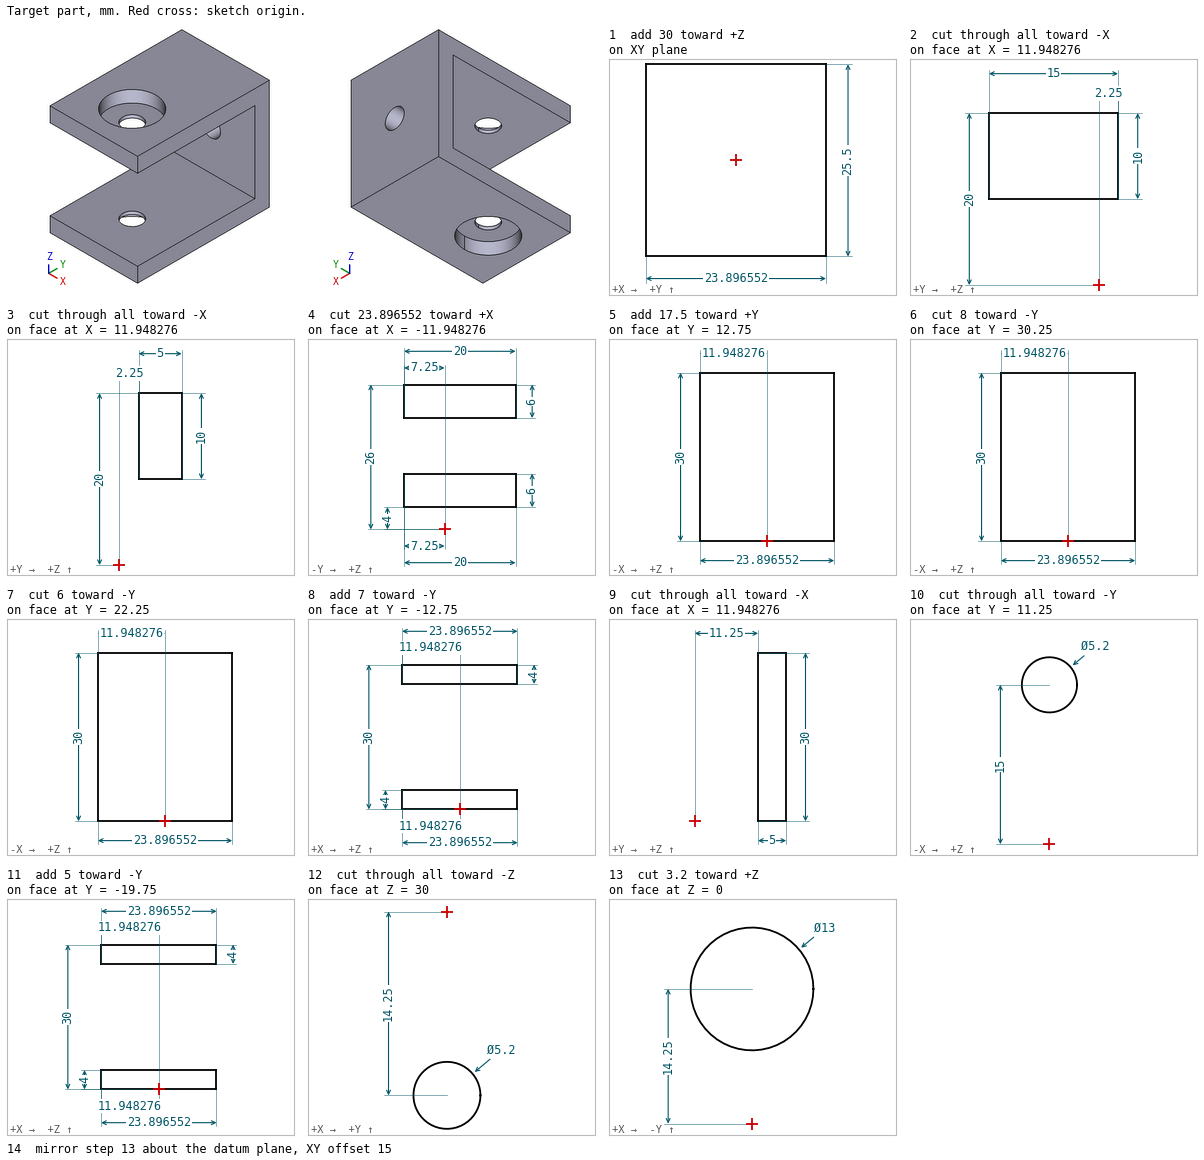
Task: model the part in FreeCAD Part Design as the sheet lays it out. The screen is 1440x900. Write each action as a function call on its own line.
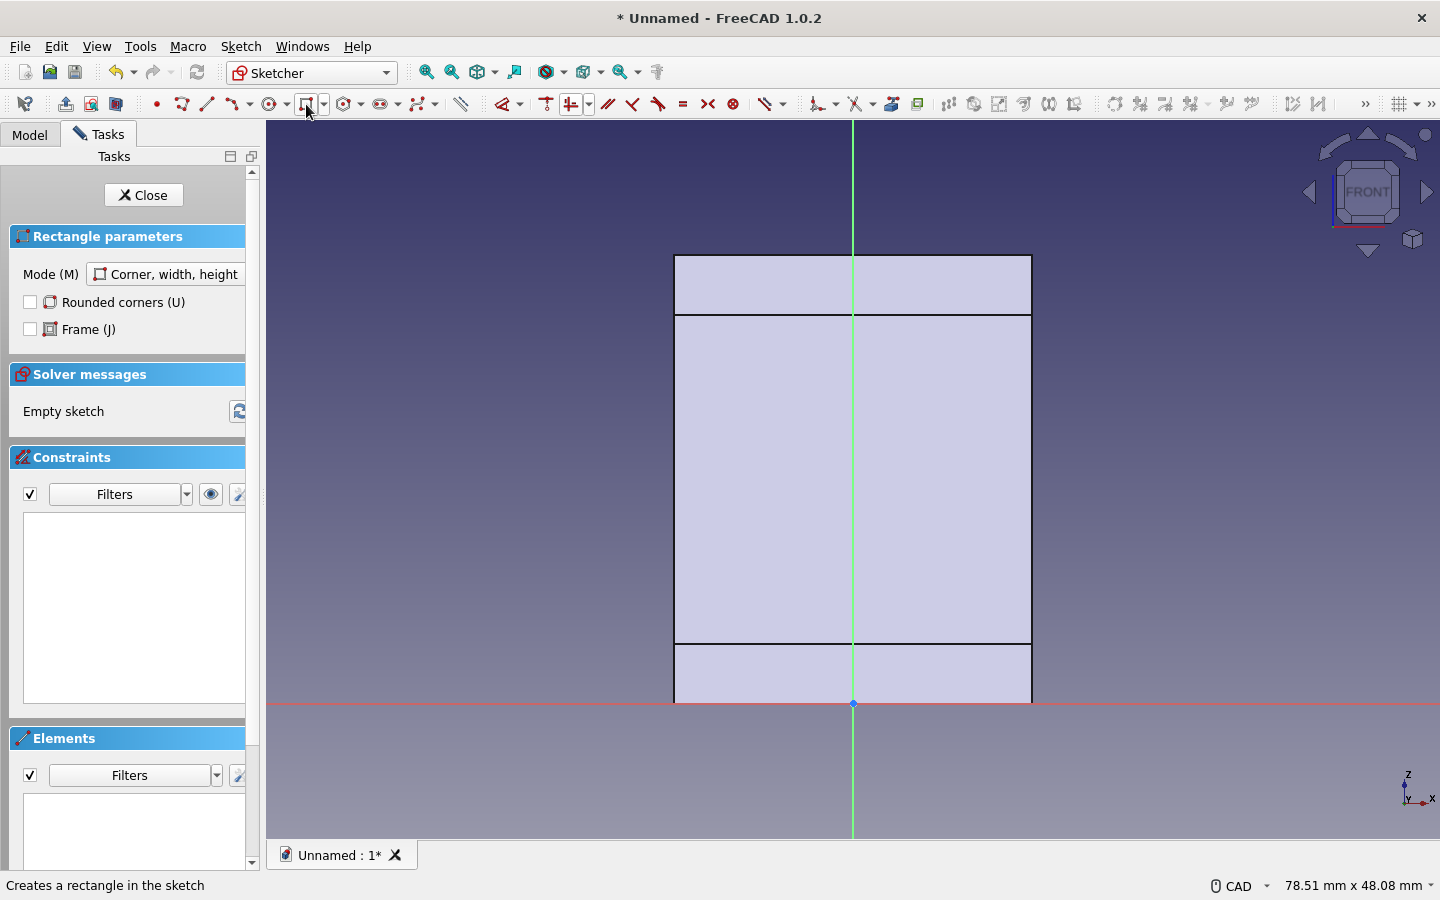
click(674, 255)
move(1032, 315)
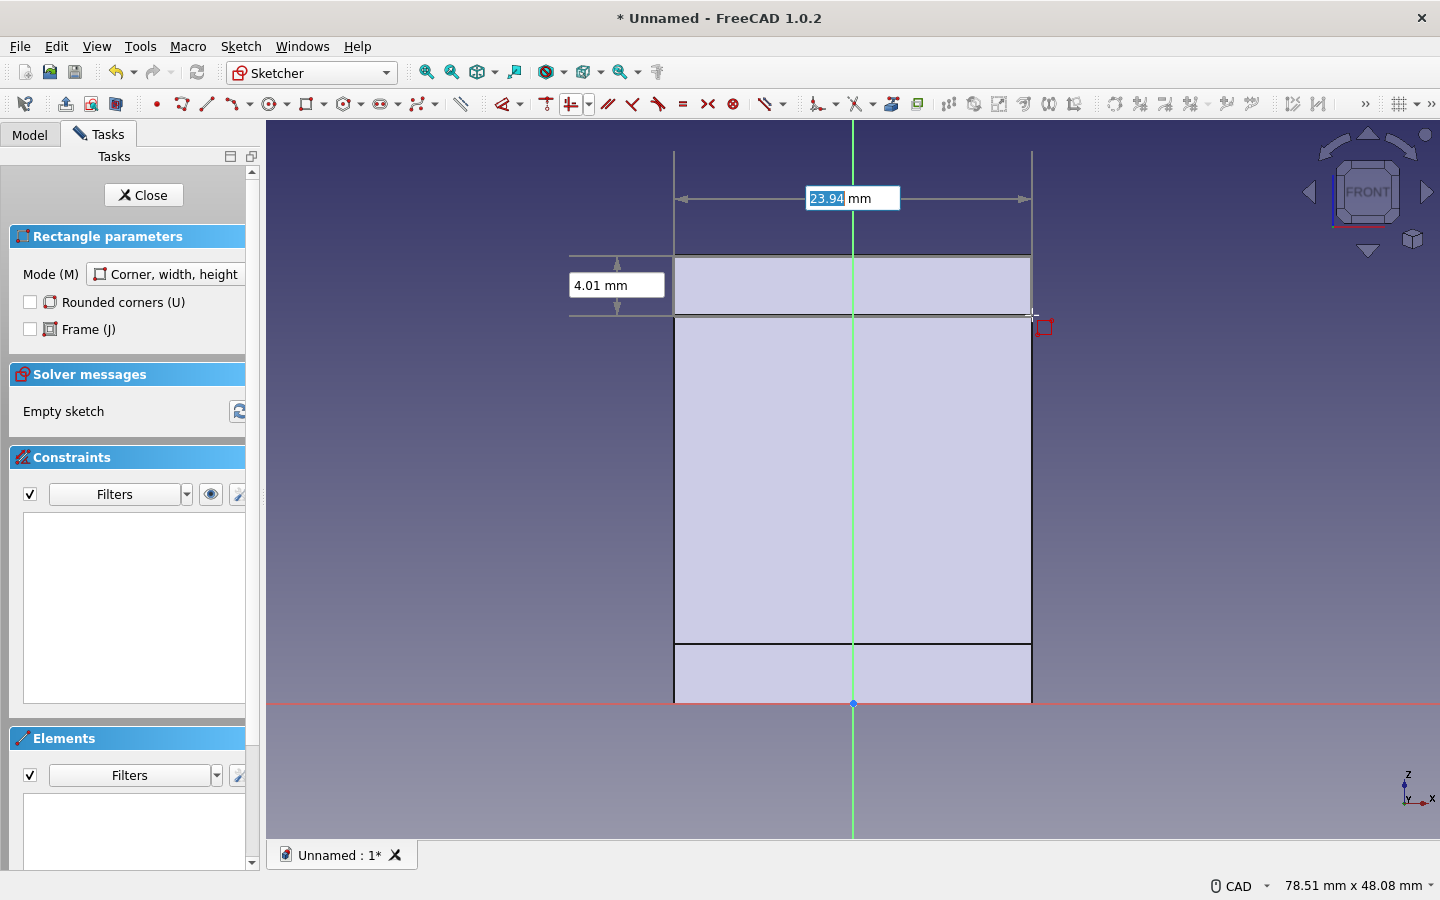
text(23.896552)
key(Tab)
text(4)
key(Return)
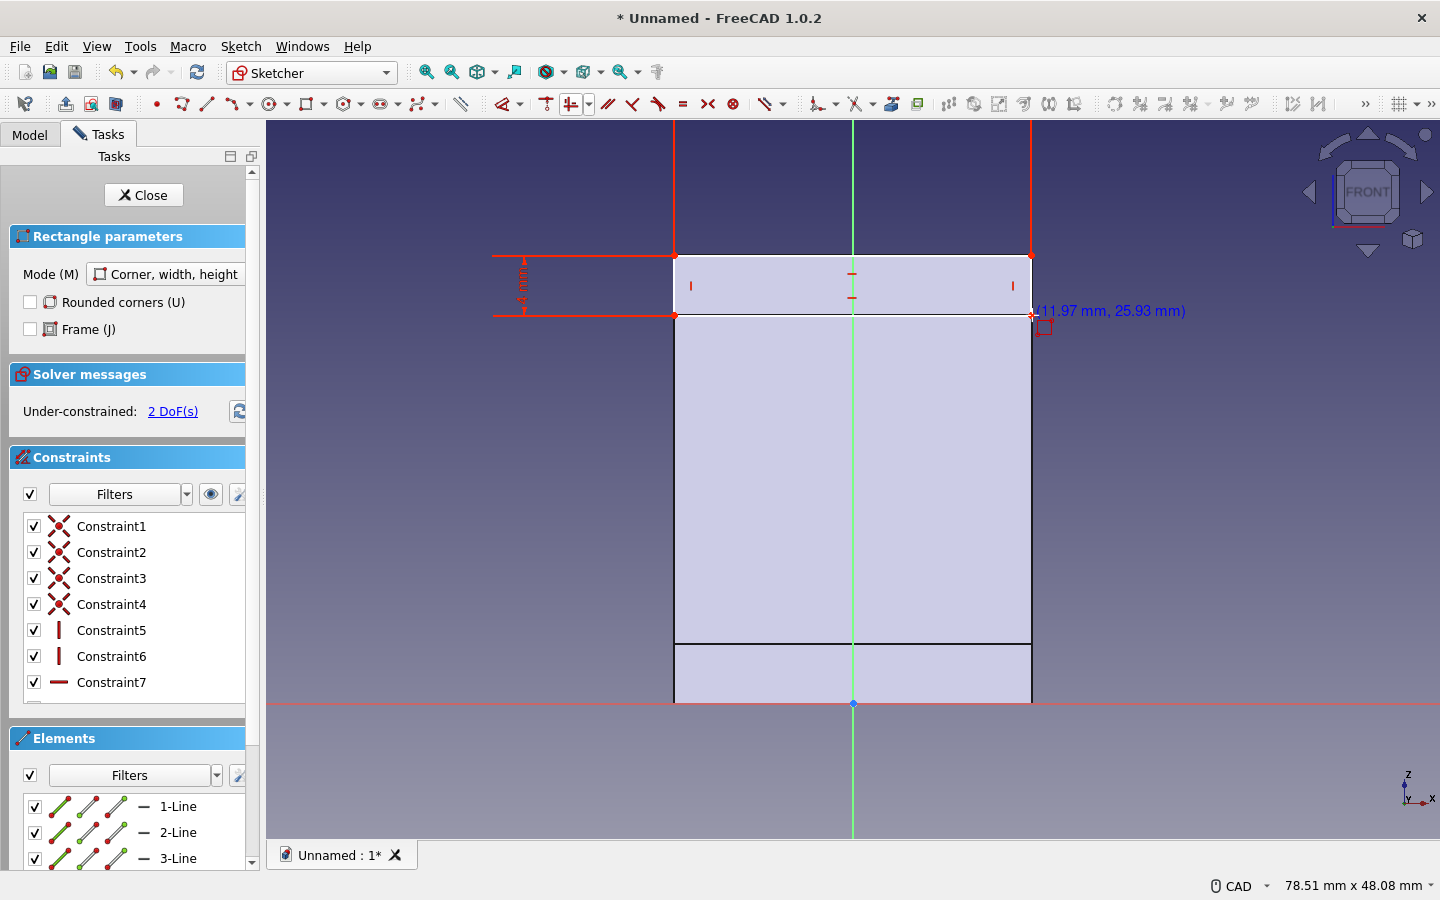
click(674, 644)
click(1032, 704)
key(Escape)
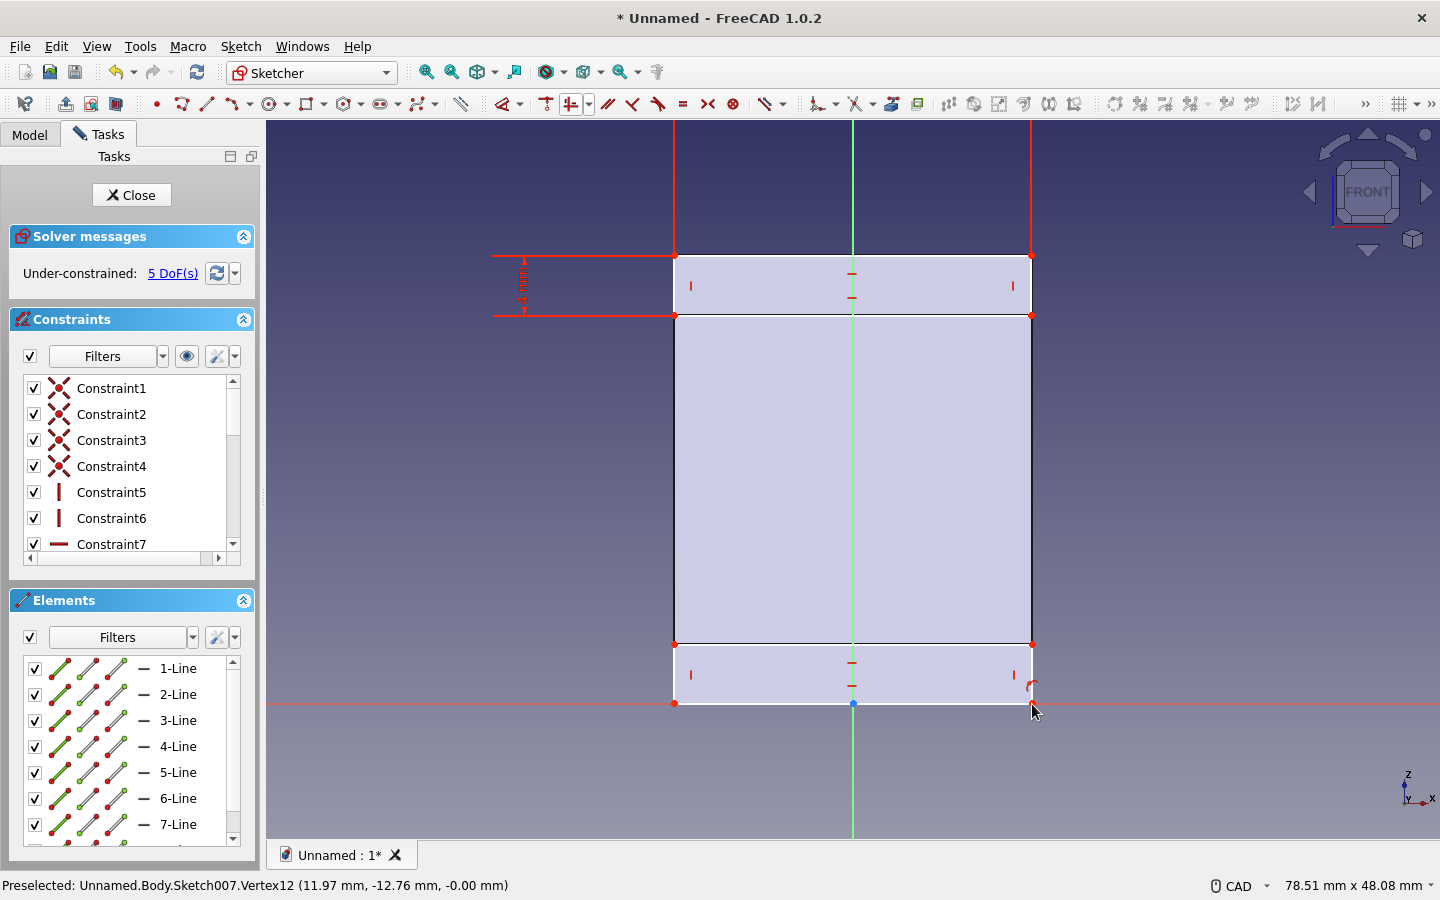
click(502, 104)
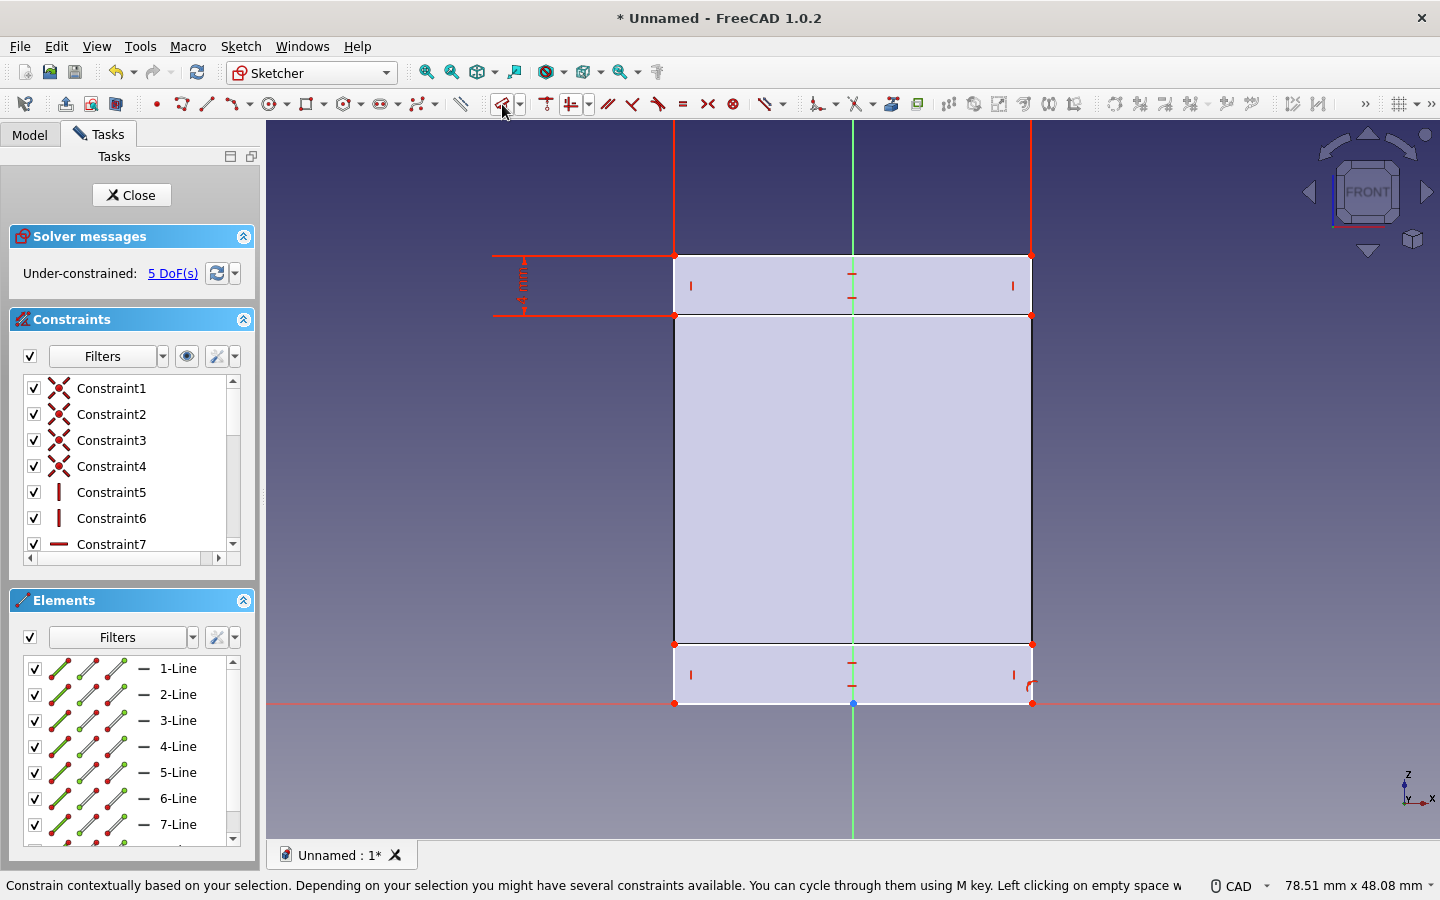
click(674, 663)
click(640, 674)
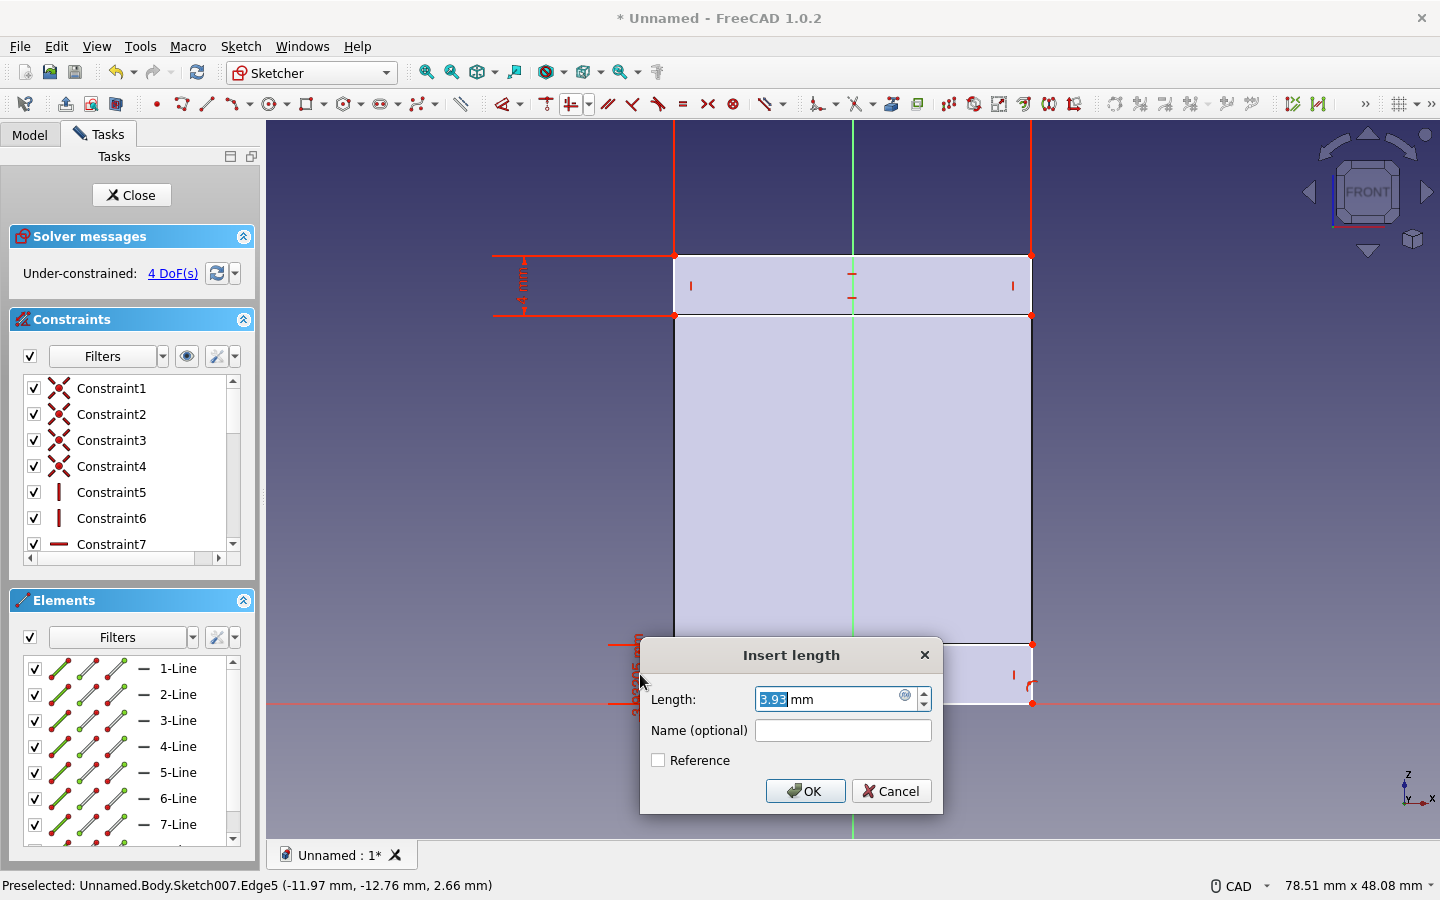
text(4)
key(Return)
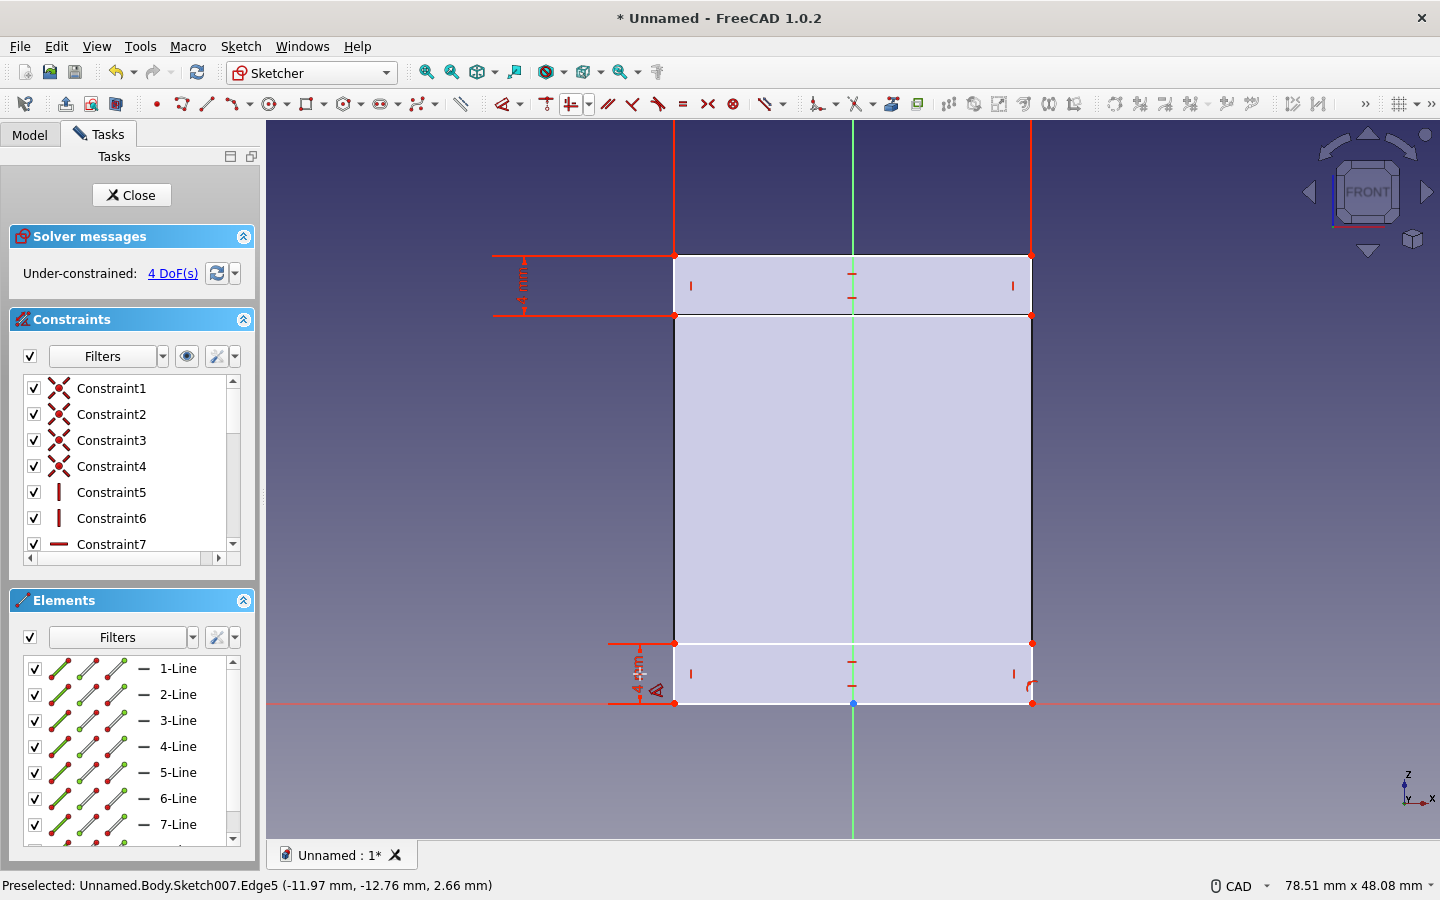
click(674, 256)
click(640, 480)